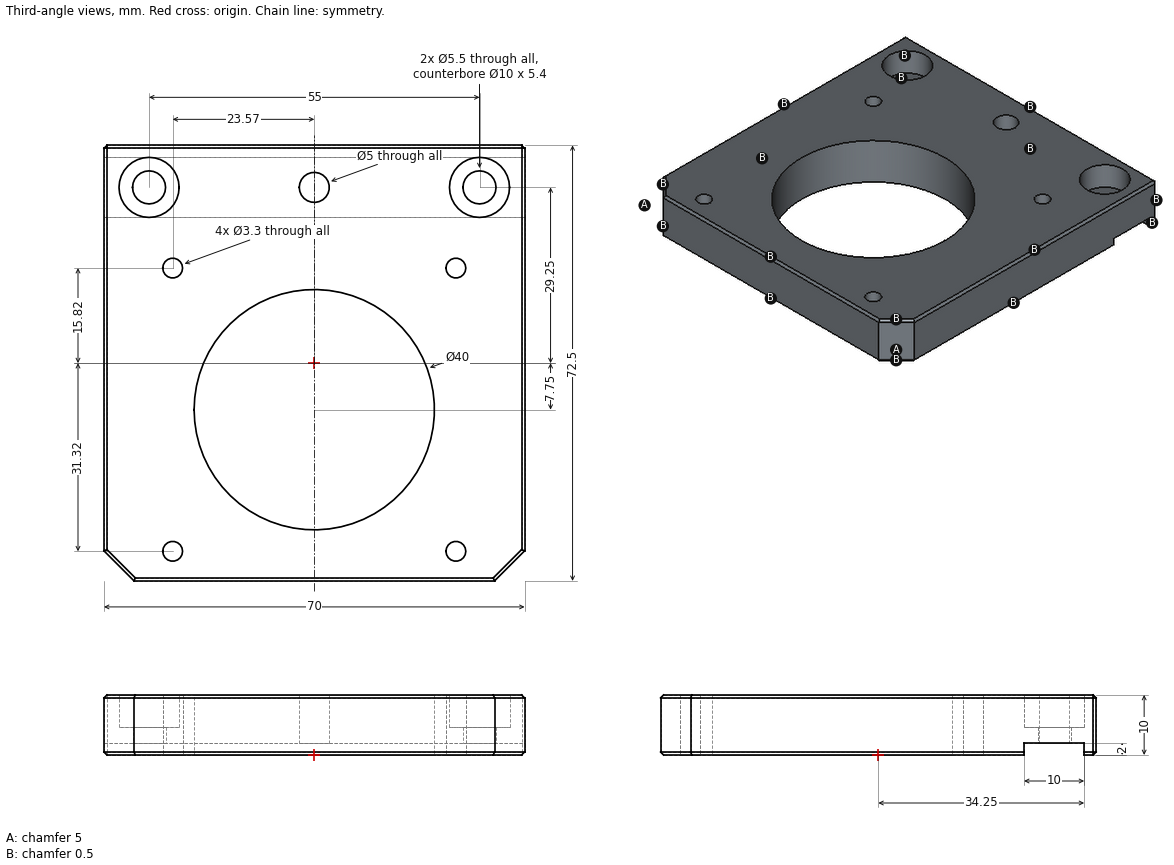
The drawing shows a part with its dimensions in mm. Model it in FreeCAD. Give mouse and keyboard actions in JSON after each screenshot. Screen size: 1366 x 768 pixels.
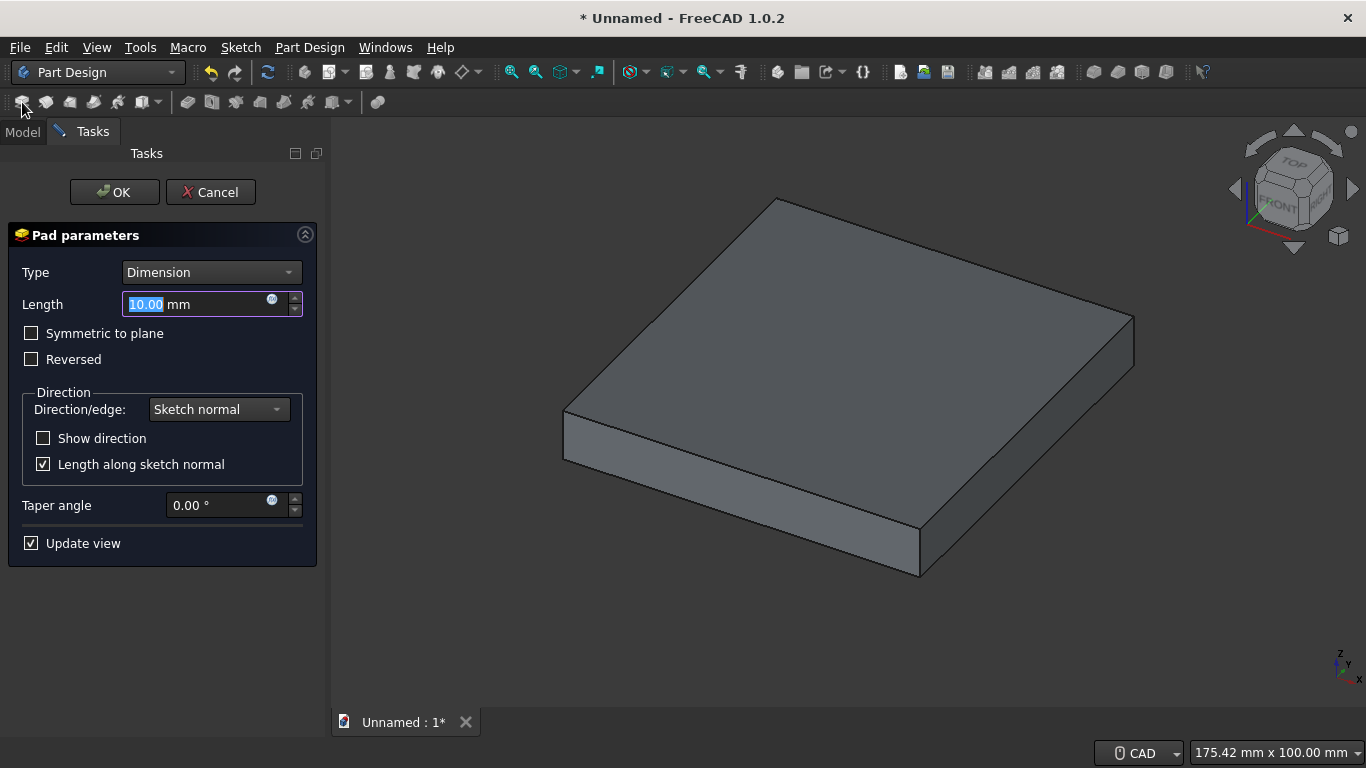
{"action": "type", "text": "10"}
{"action": "key", "text": "Tab"}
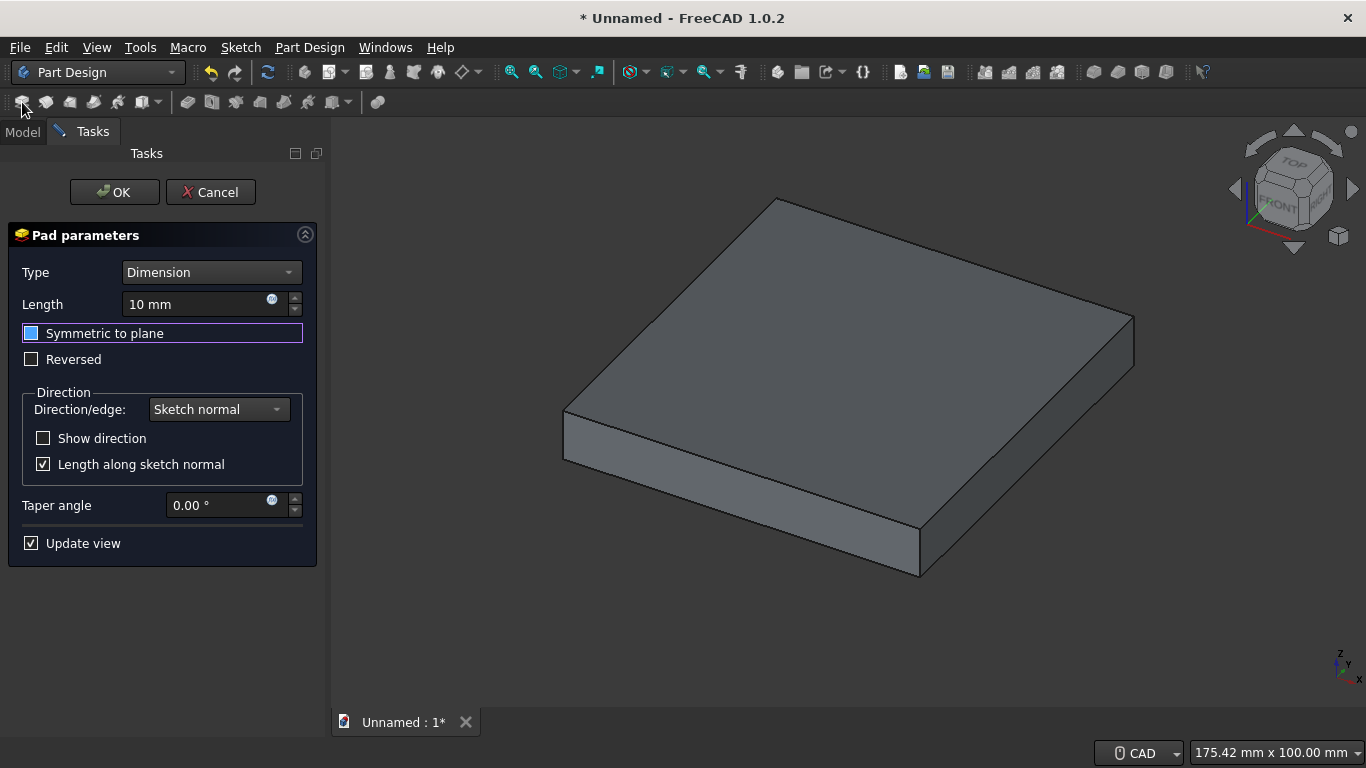
{"action": "left_click", "coordinate": [115, 192]}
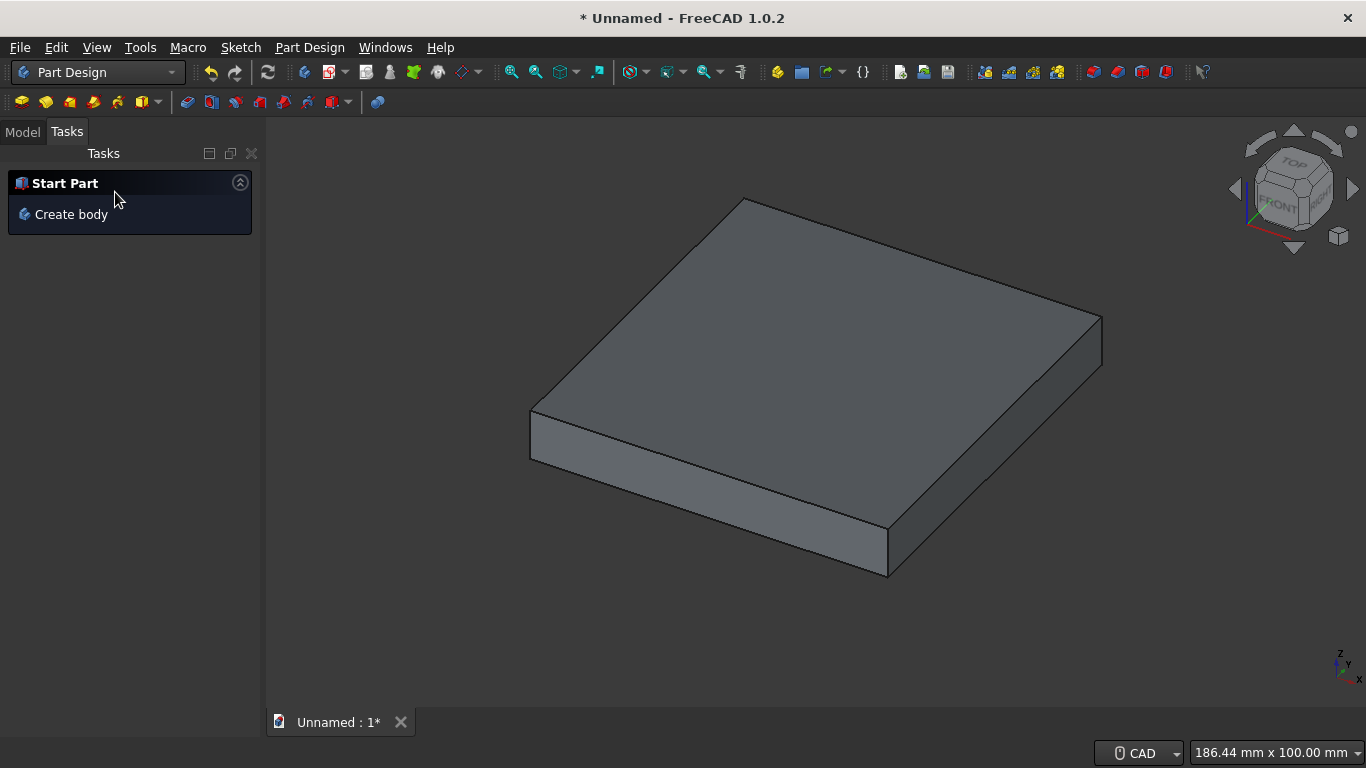
{"action": "key", "text": "6"}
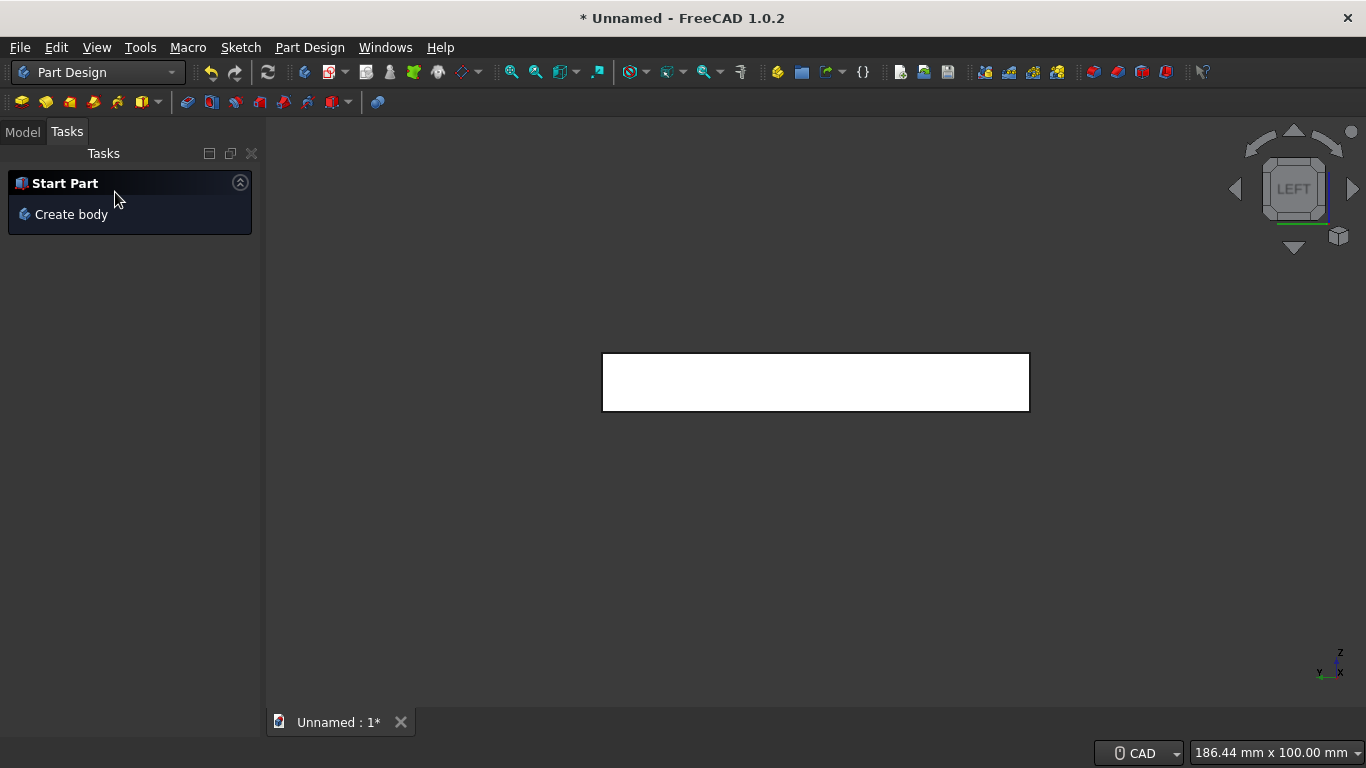
{"action": "left_click", "coordinate": [512, 72]}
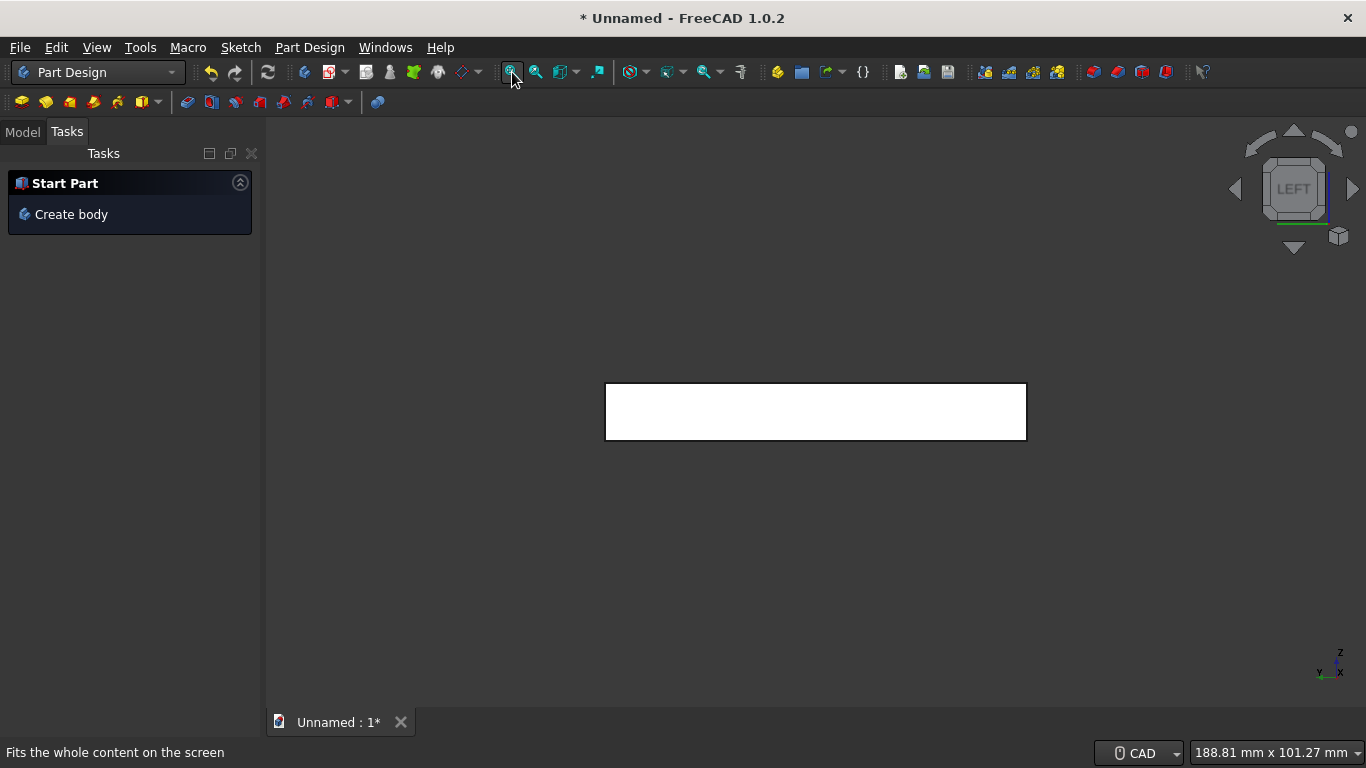
{"action": "left_click", "coordinate": [635, 411]}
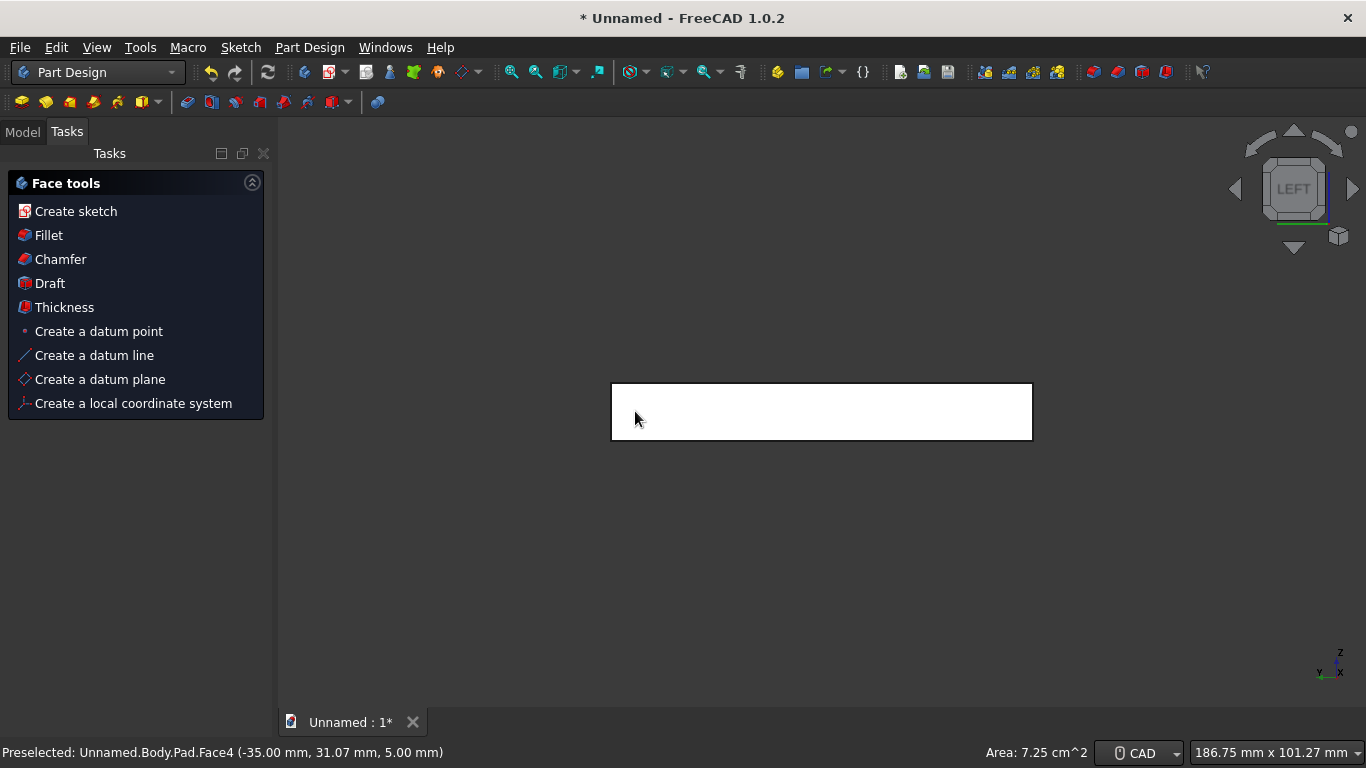
{"action": "left_click", "coordinate": [330, 72]}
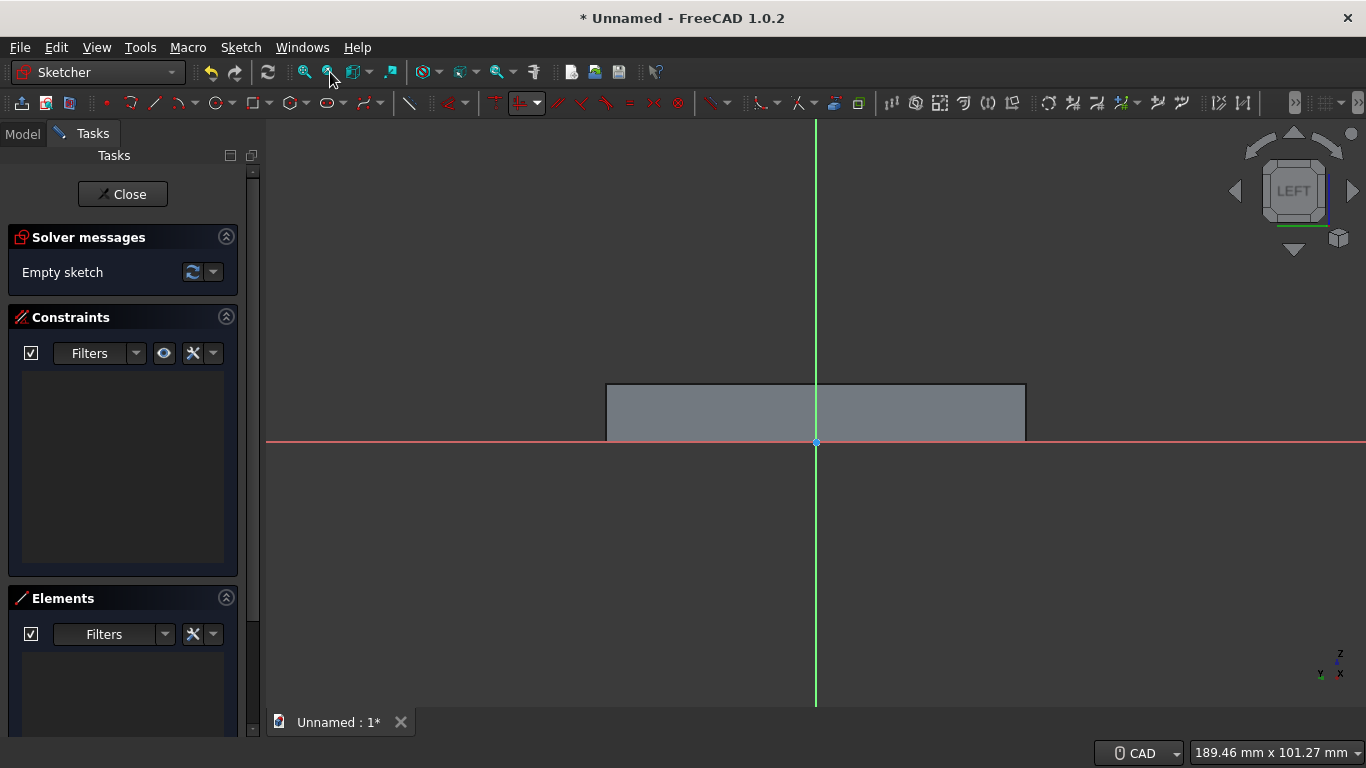
{"action": "scroll", "coordinate": [636, 439], "scroll_direction": "up", "scroll_amount": 12}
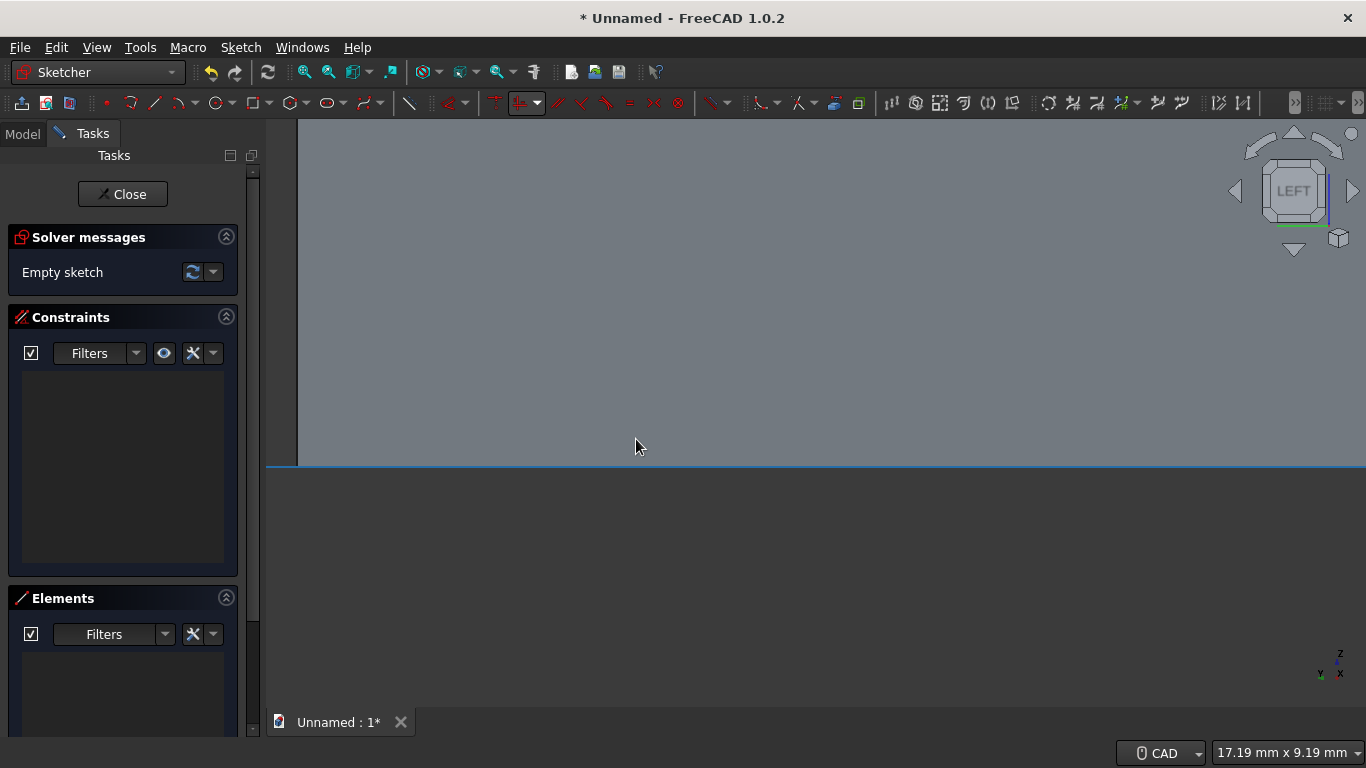
{"action": "key", "text": "g r"}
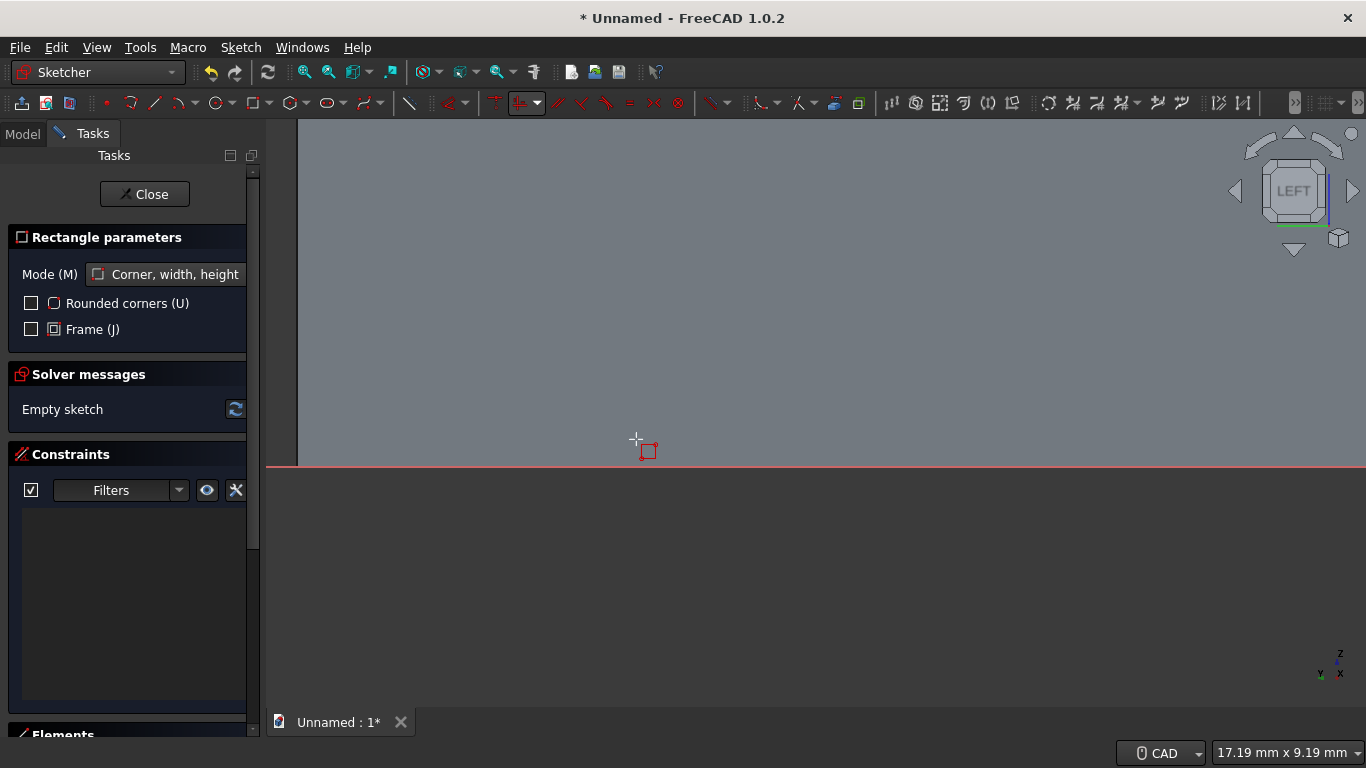
{"action": "left_click", "coordinate": [425, 339]}
{"action": "left_click", "coordinate": [1065, 467]}
{"action": "key", "text": "Escape"}